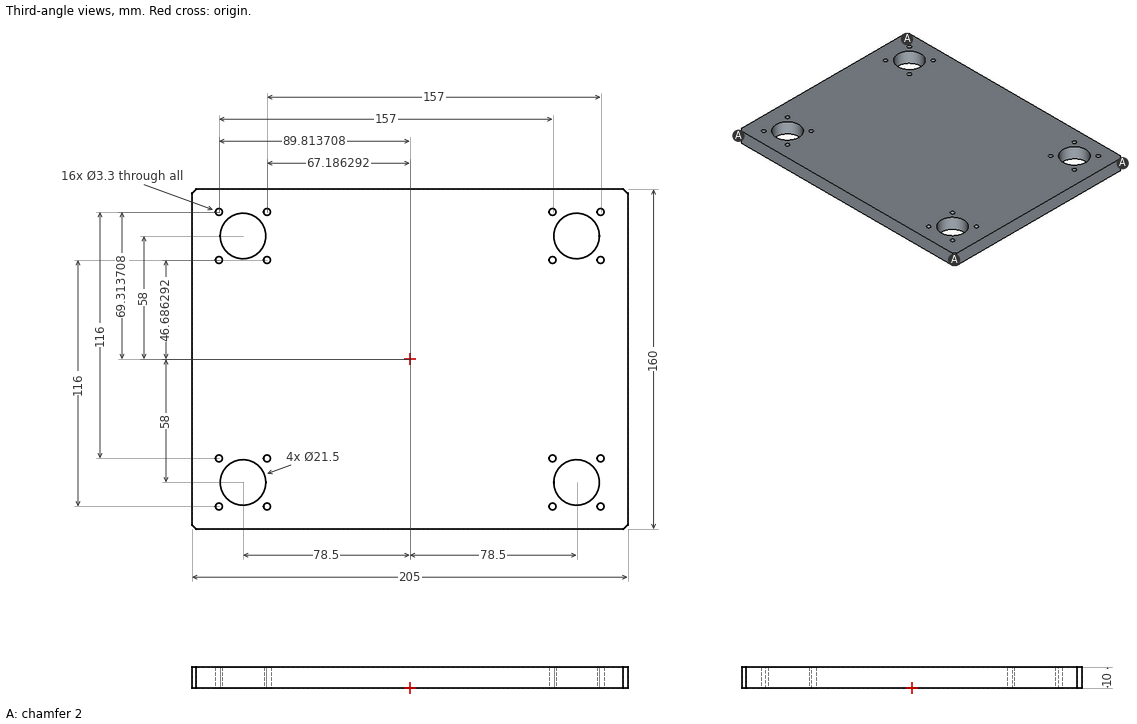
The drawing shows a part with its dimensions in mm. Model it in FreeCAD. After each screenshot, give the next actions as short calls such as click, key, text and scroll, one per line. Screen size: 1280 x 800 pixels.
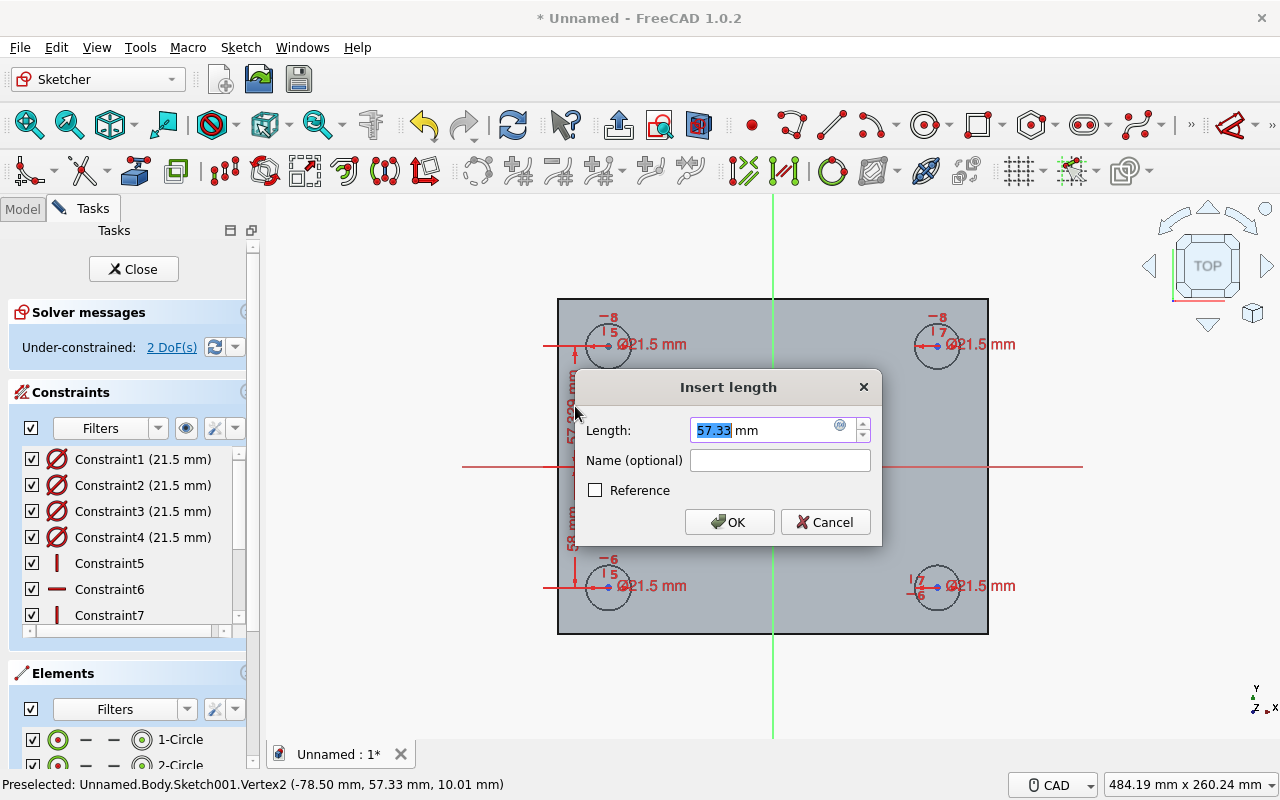
text(58)
key(Return)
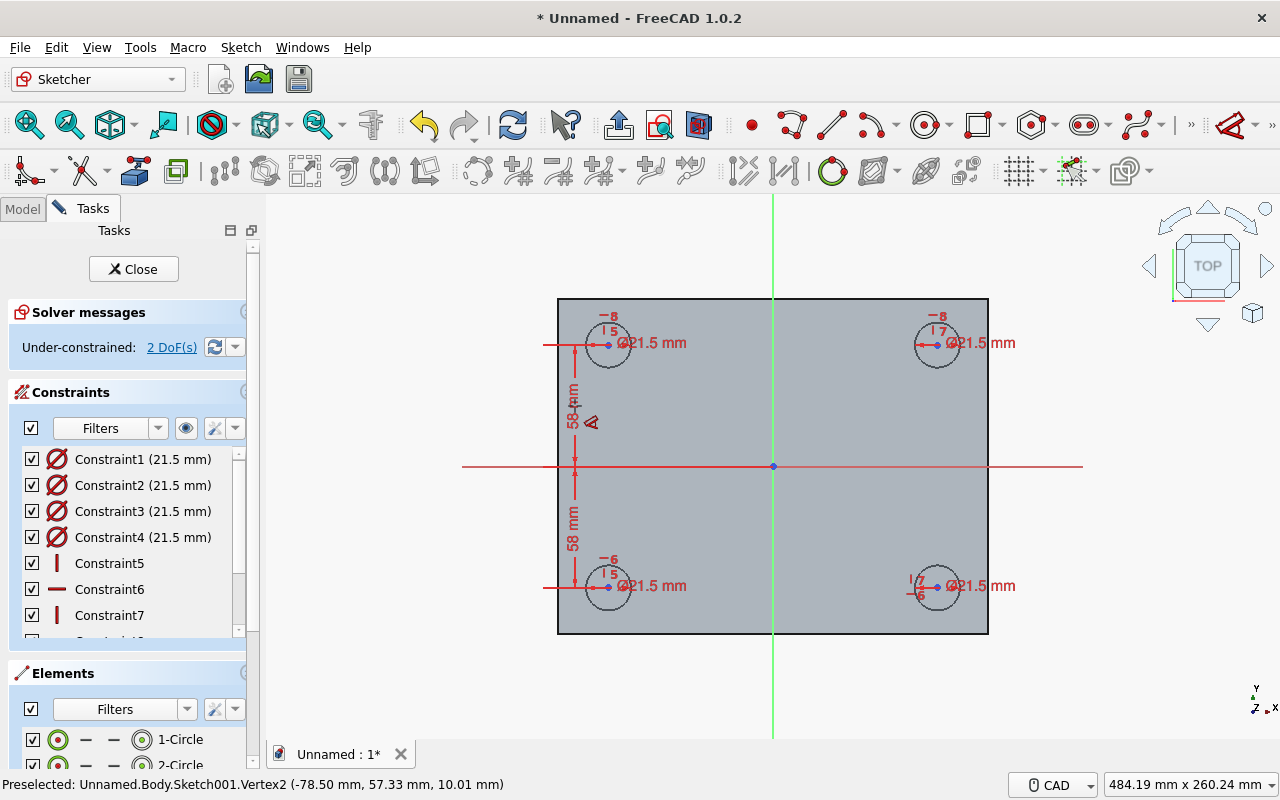
click(609, 588)
click(691, 622)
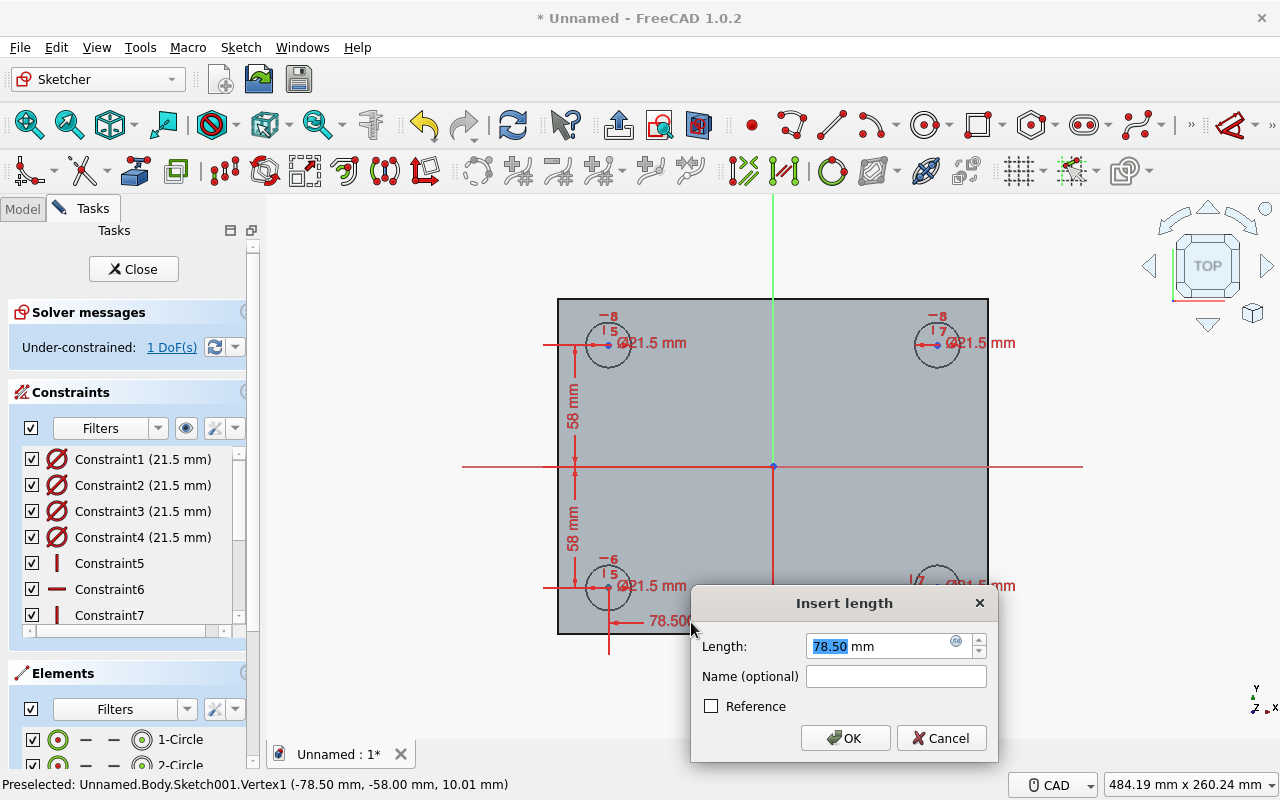
text(78.5)
key(Return)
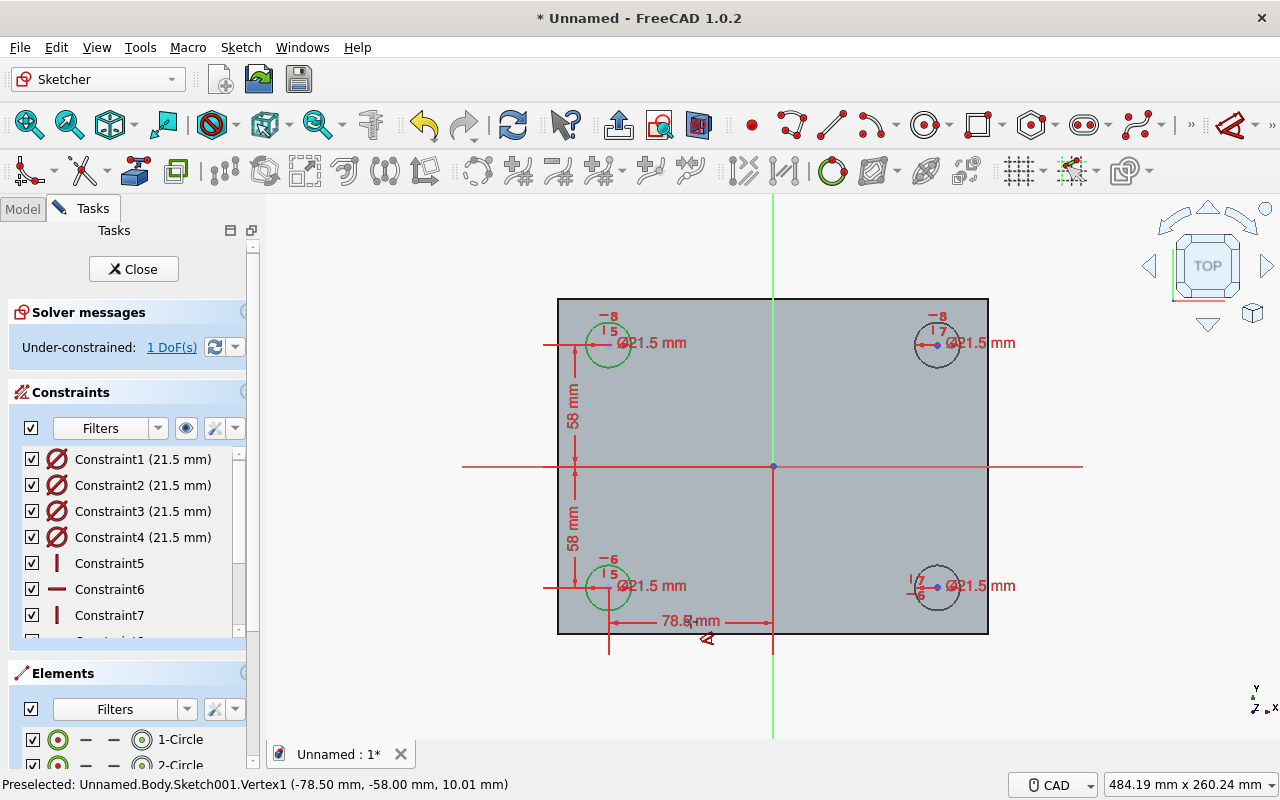
click(937, 588)
click(855, 622)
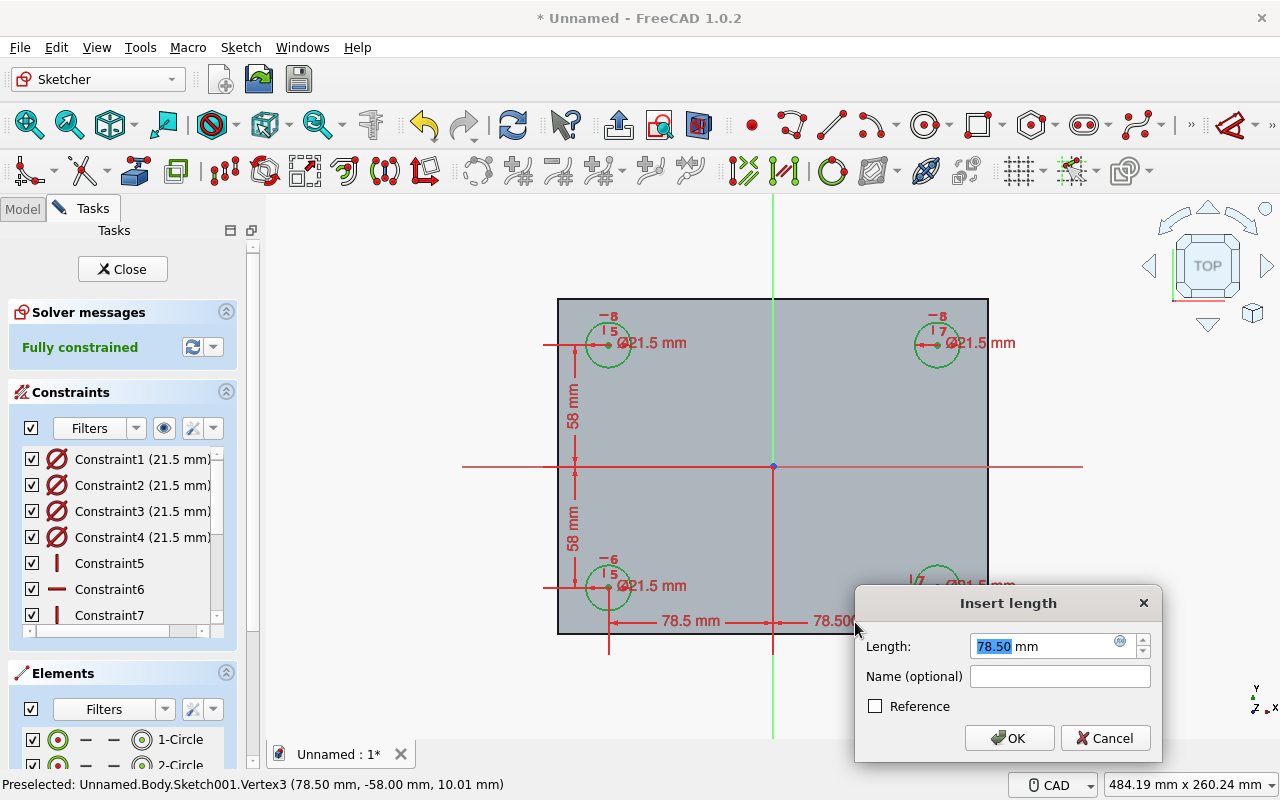
text(78.5)
key(Return)
key(Escape)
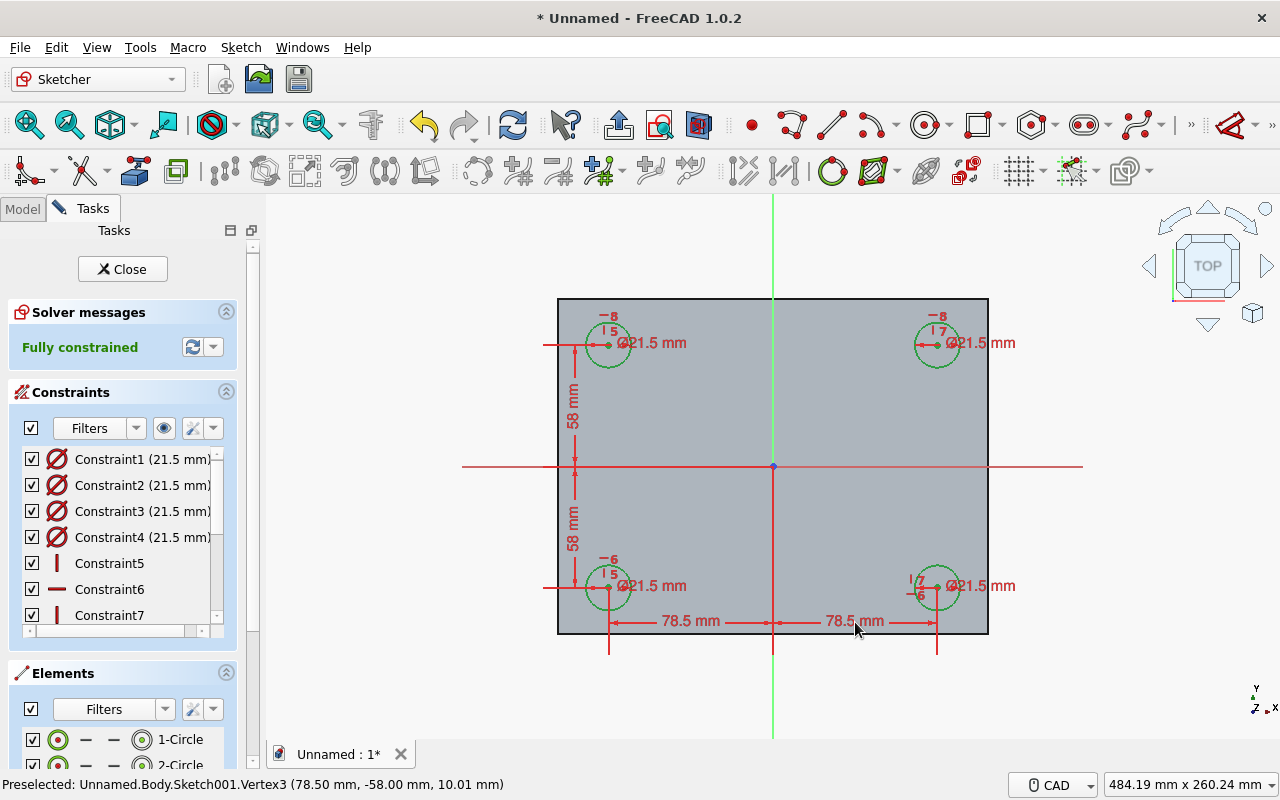
click(123, 269)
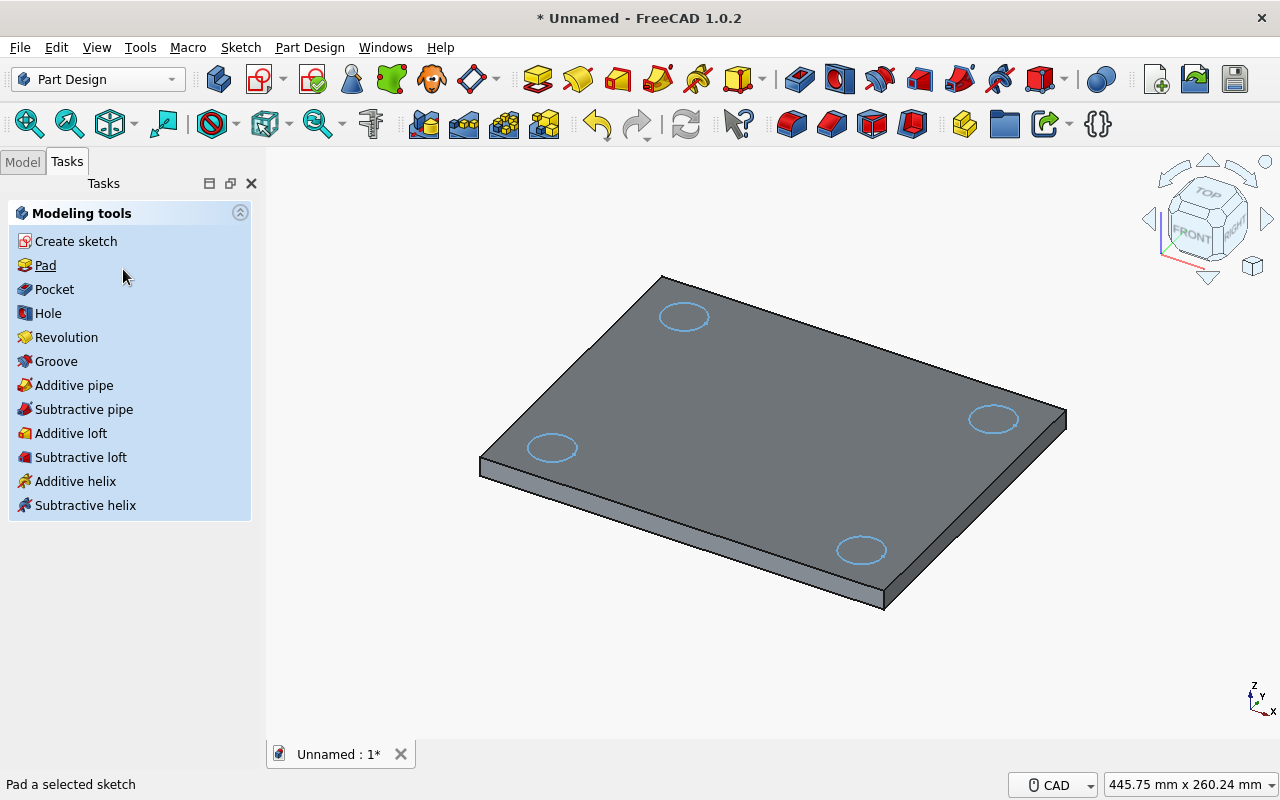
click(800, 80)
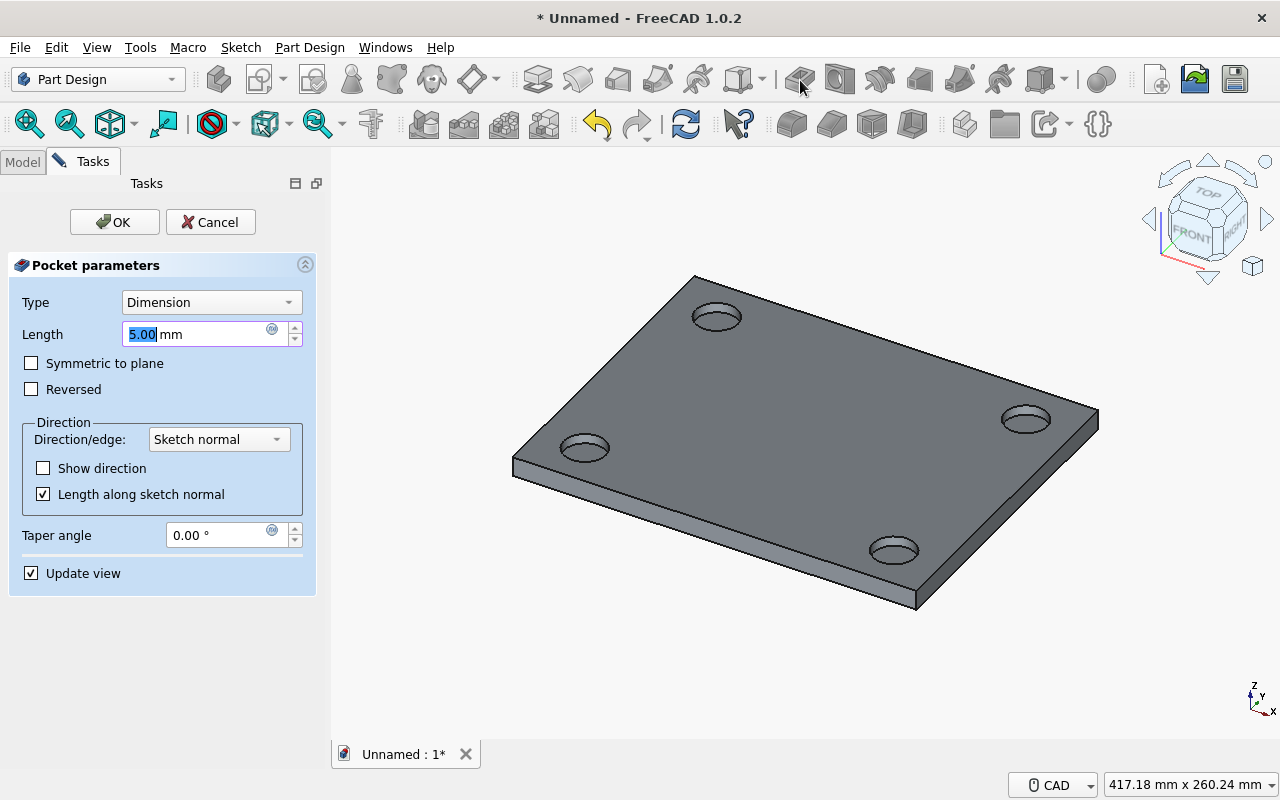
click(212, 302)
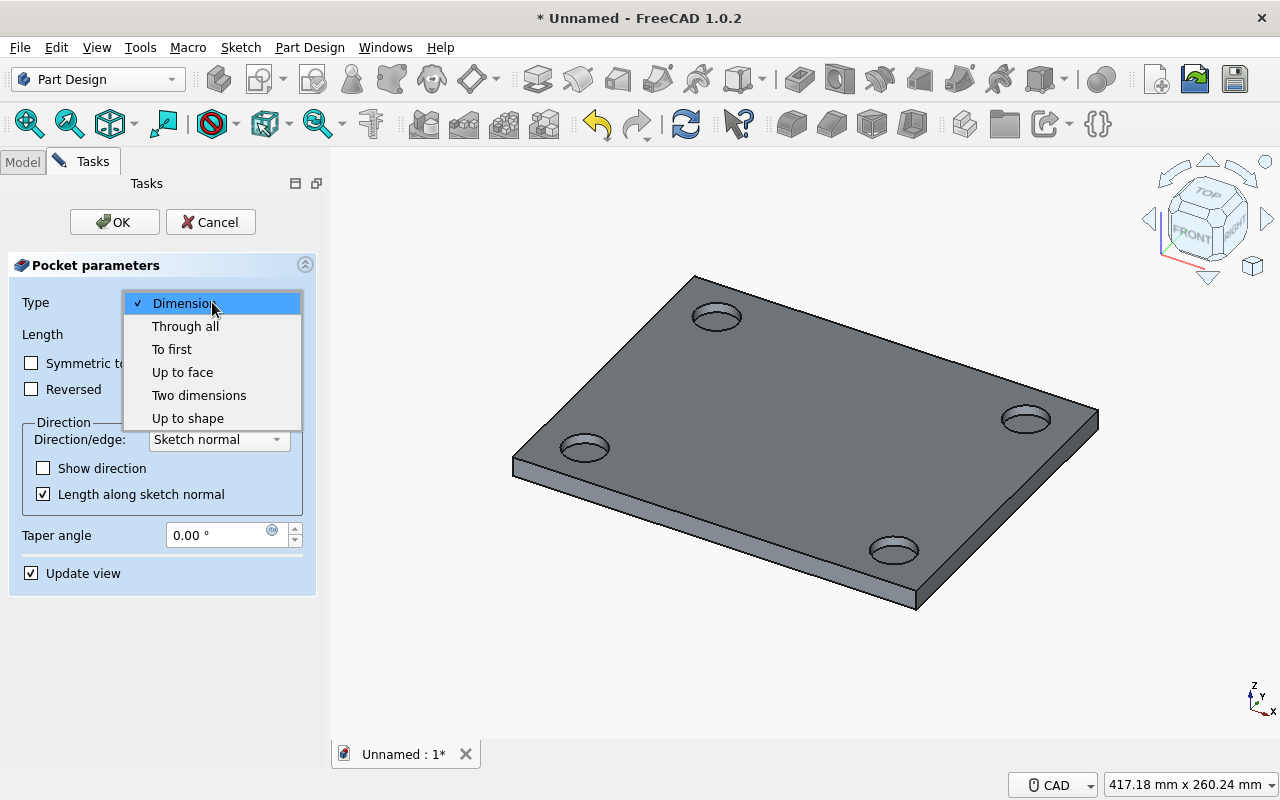
click(212, 326)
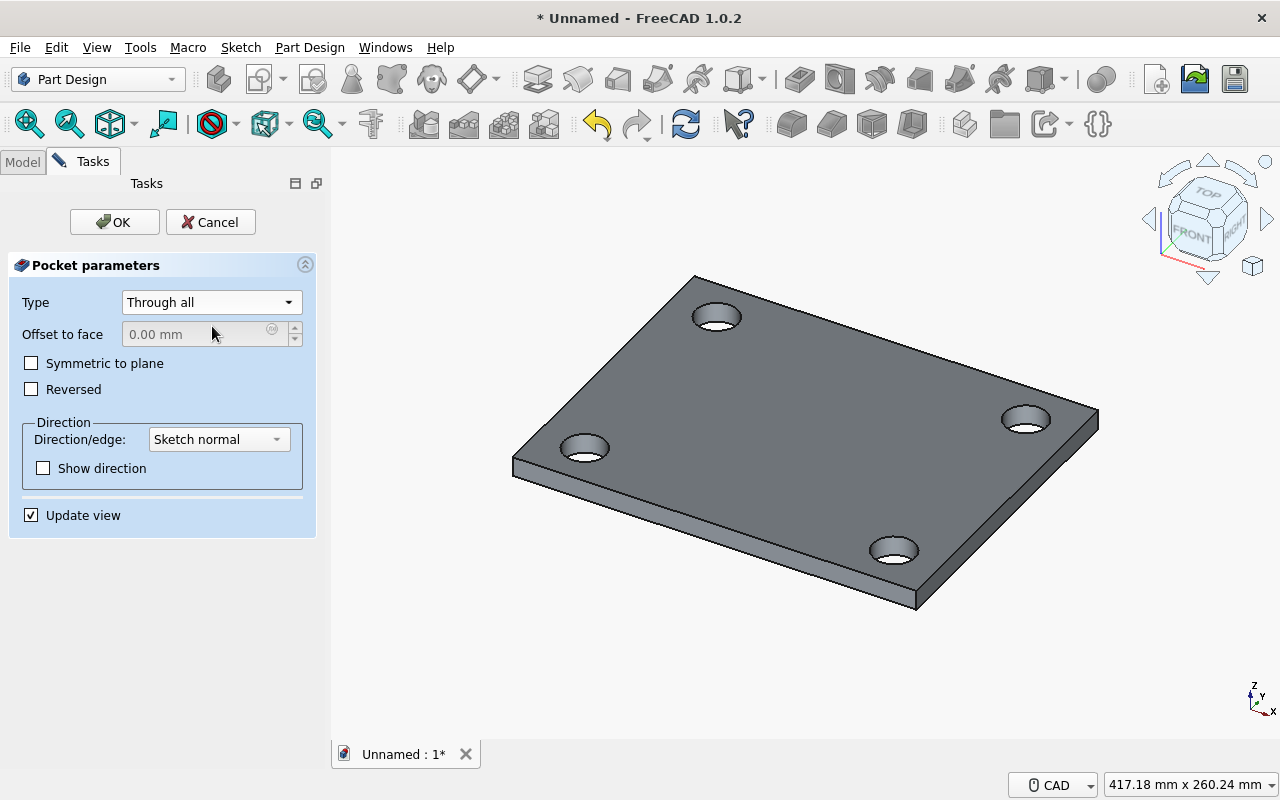
click(115, 222)